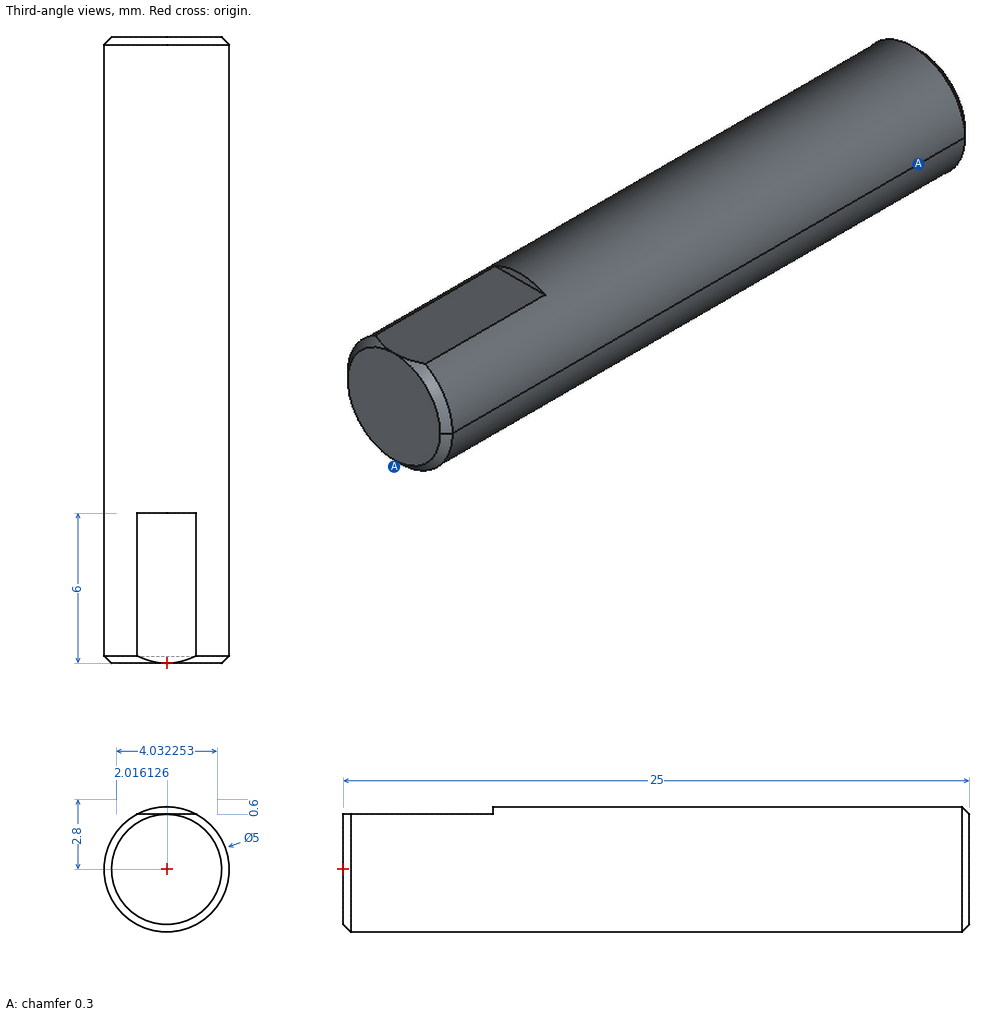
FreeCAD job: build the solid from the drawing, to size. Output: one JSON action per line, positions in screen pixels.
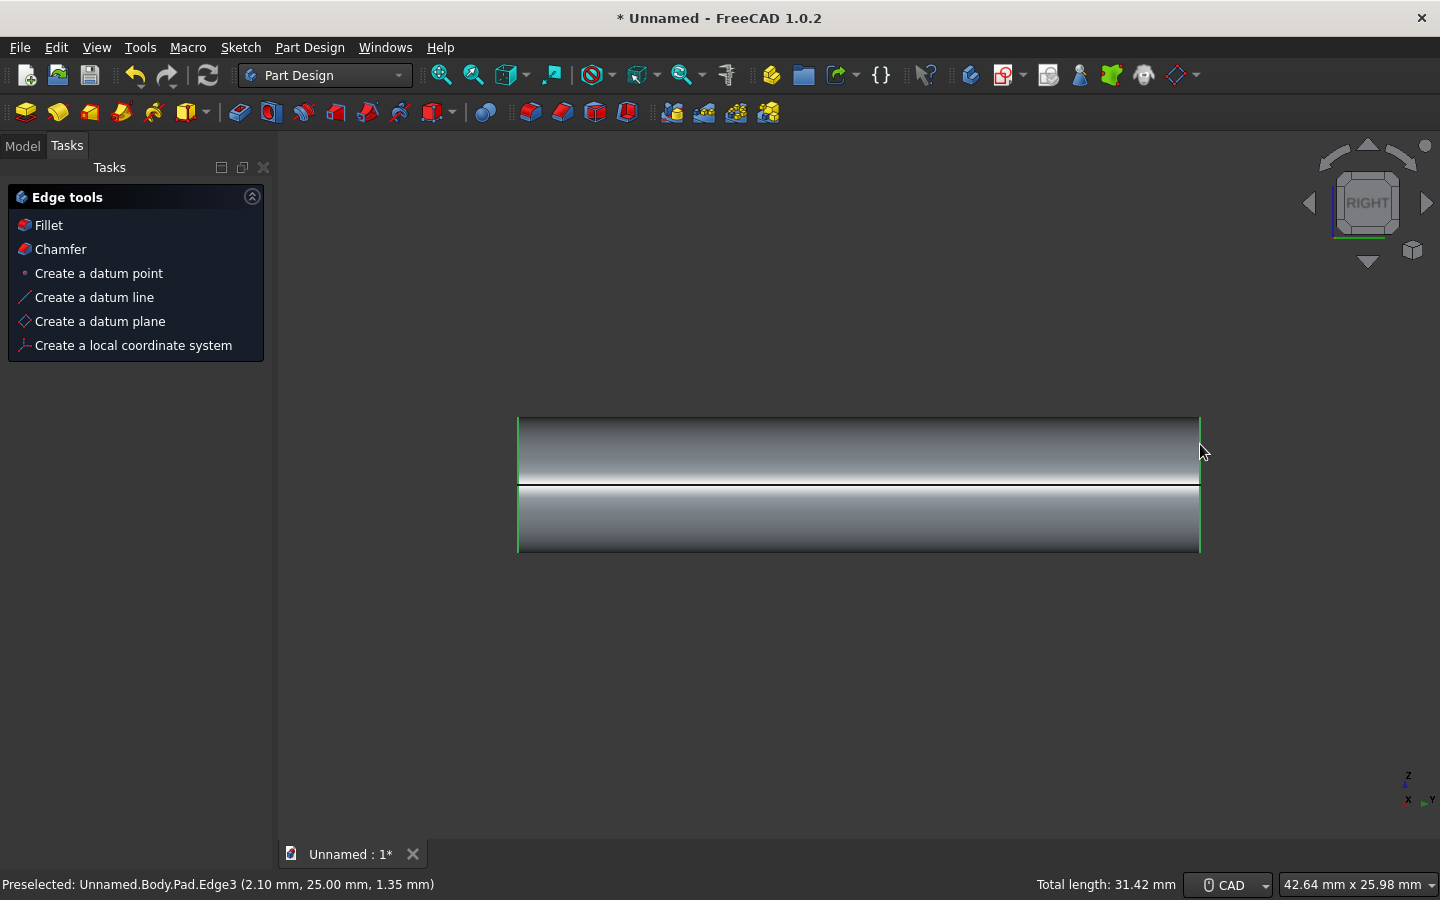
{"action": "left_click", "coordinate": [564, 112]}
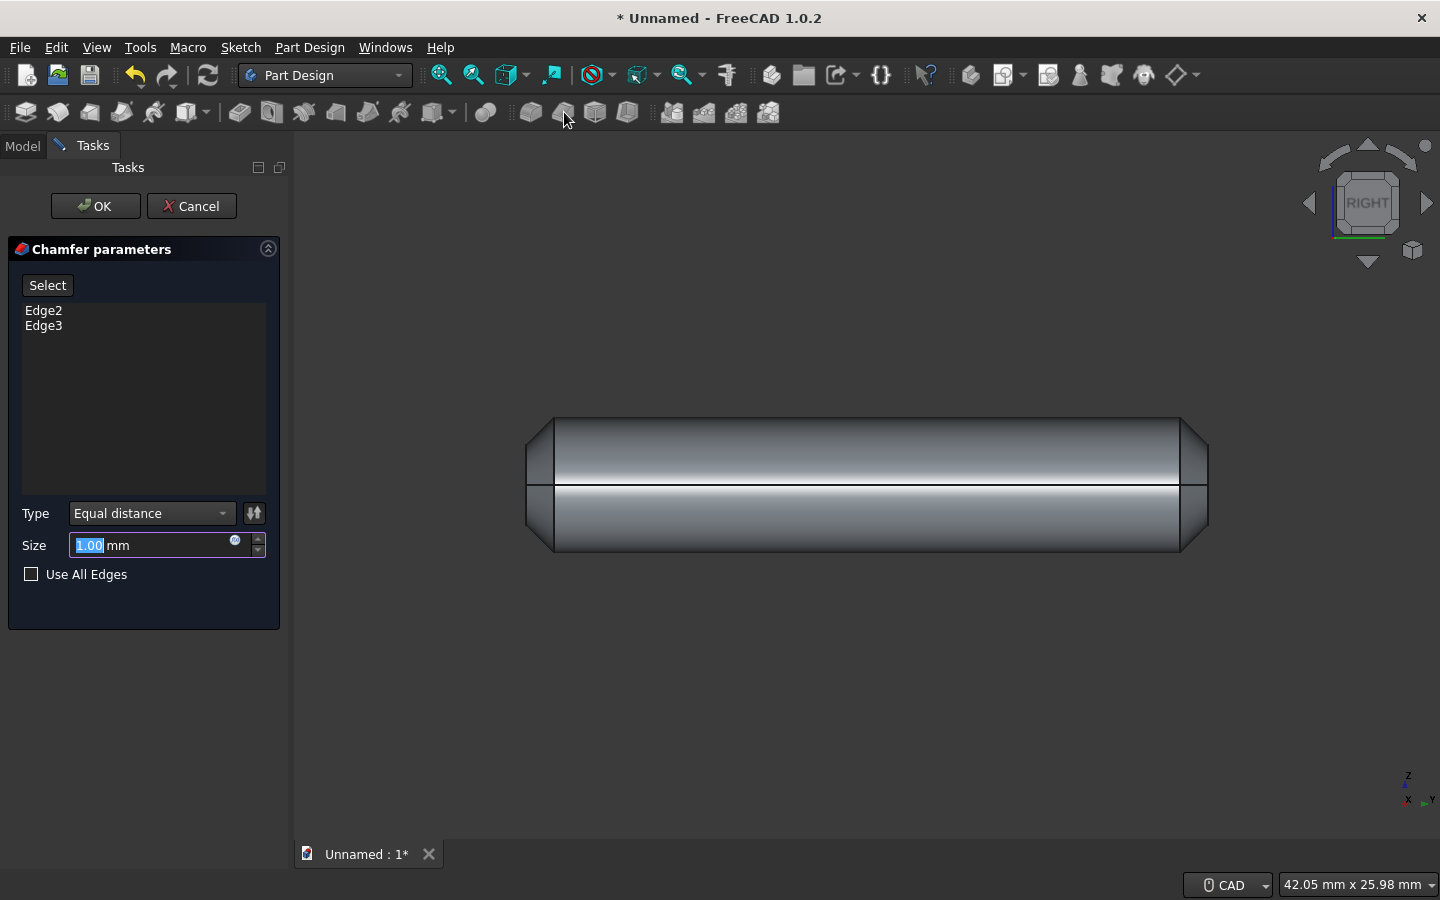
{"action": "type", "text": "0.3"}
{"action": "key", "text": "Tab"}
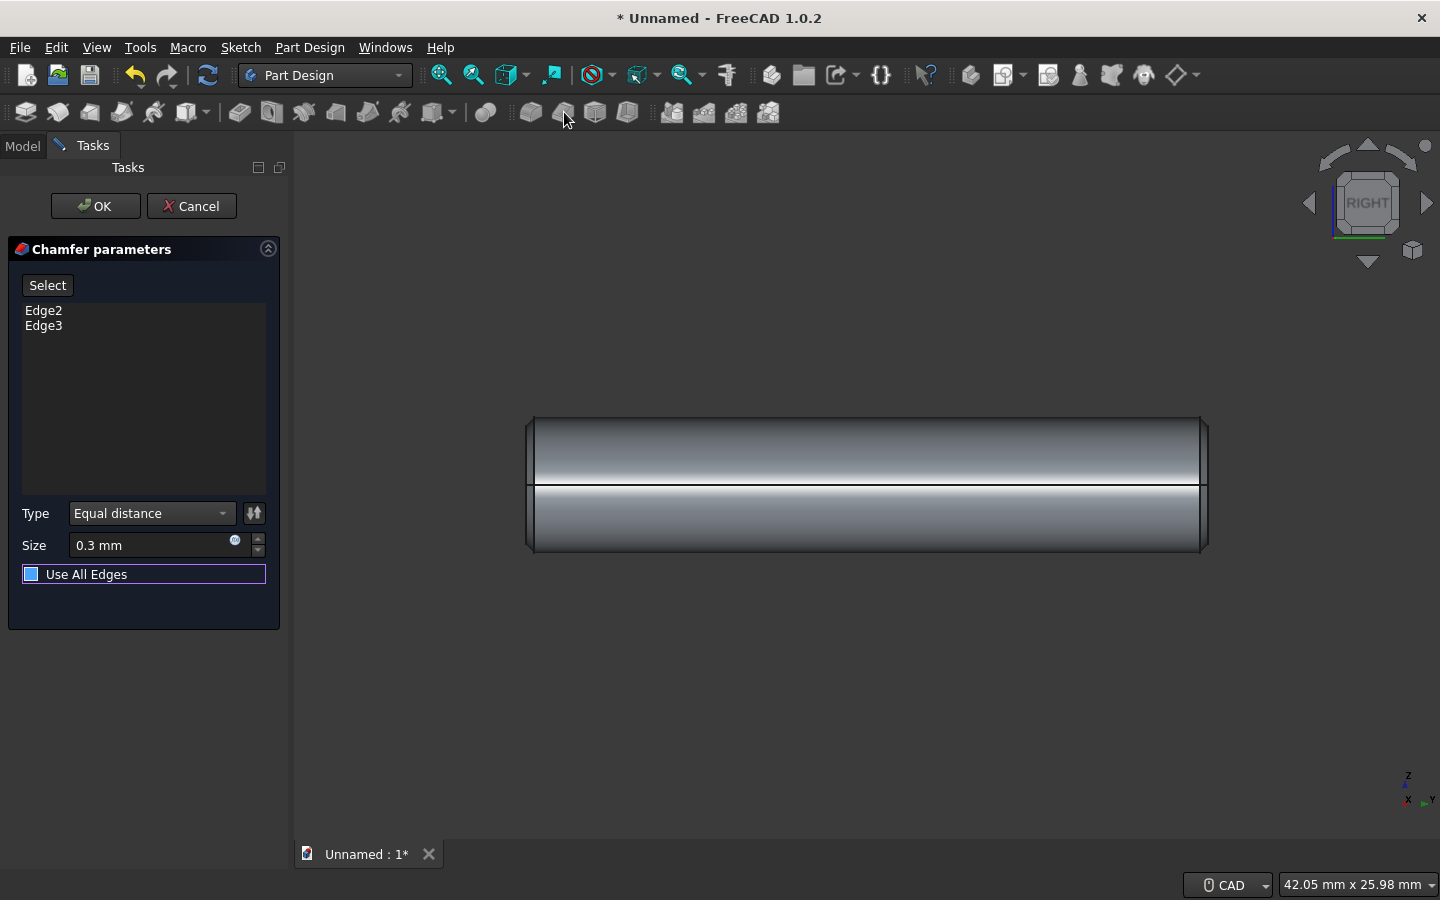
{"action": "left_click", "coordinate": [96, 206]}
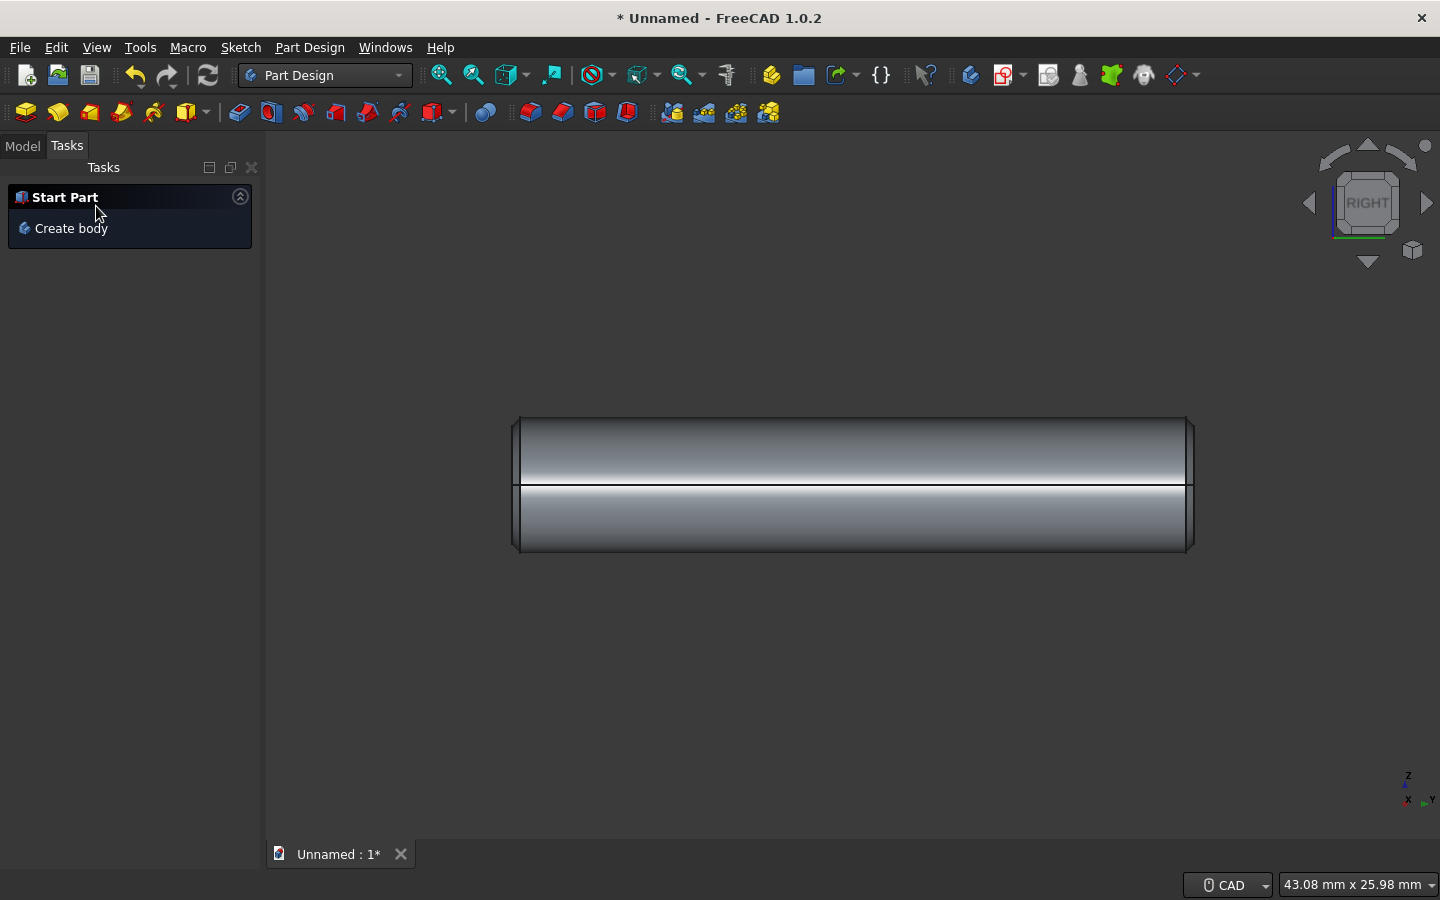
{"action": "left_click", "coordinate": [1004, 76]}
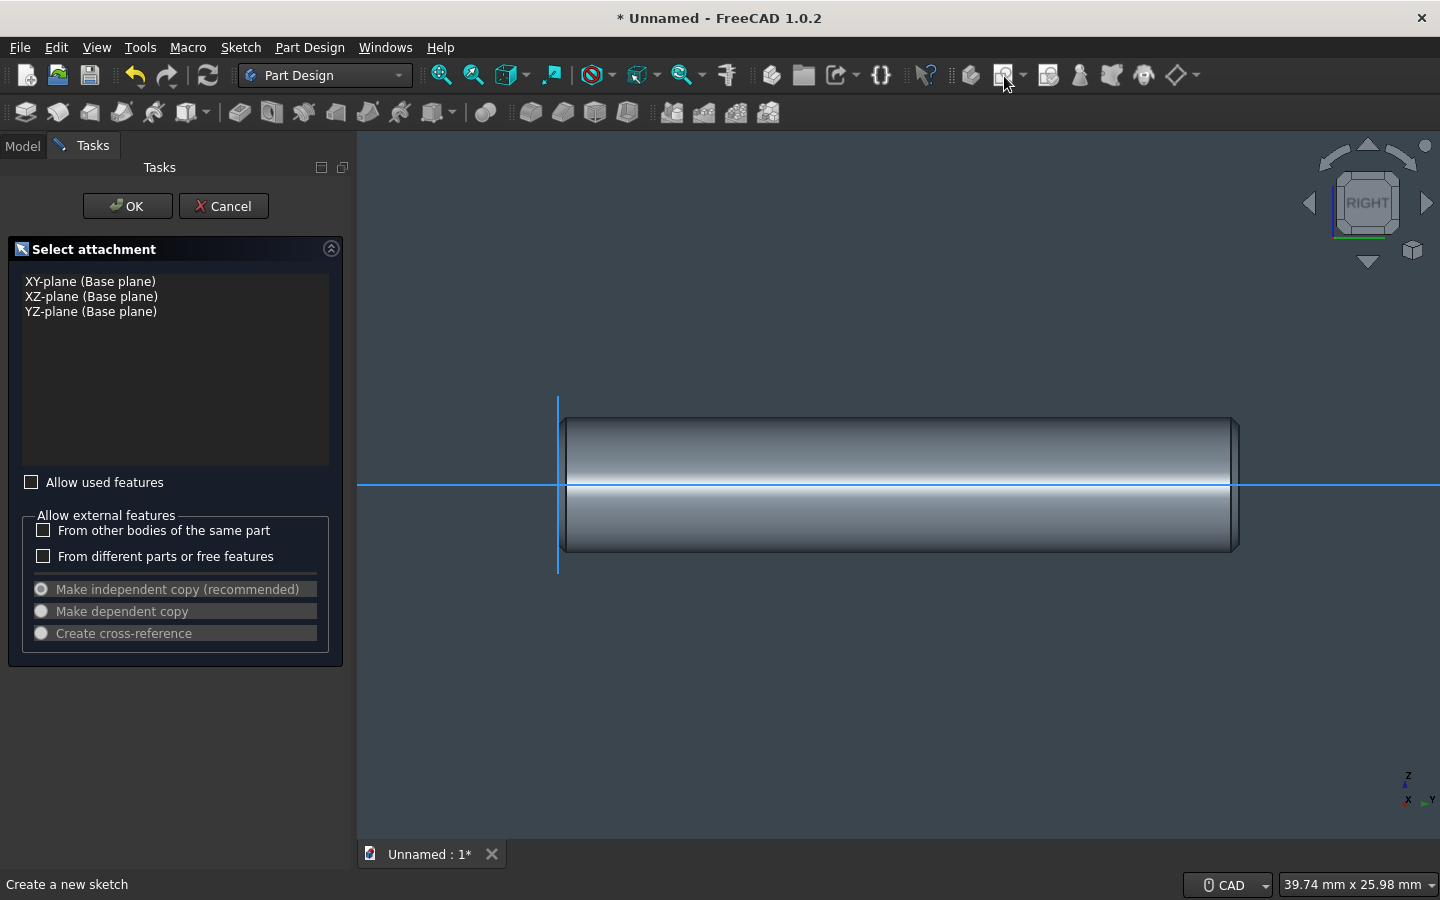
{"action": "left_click", "coordinate": [82, 296]}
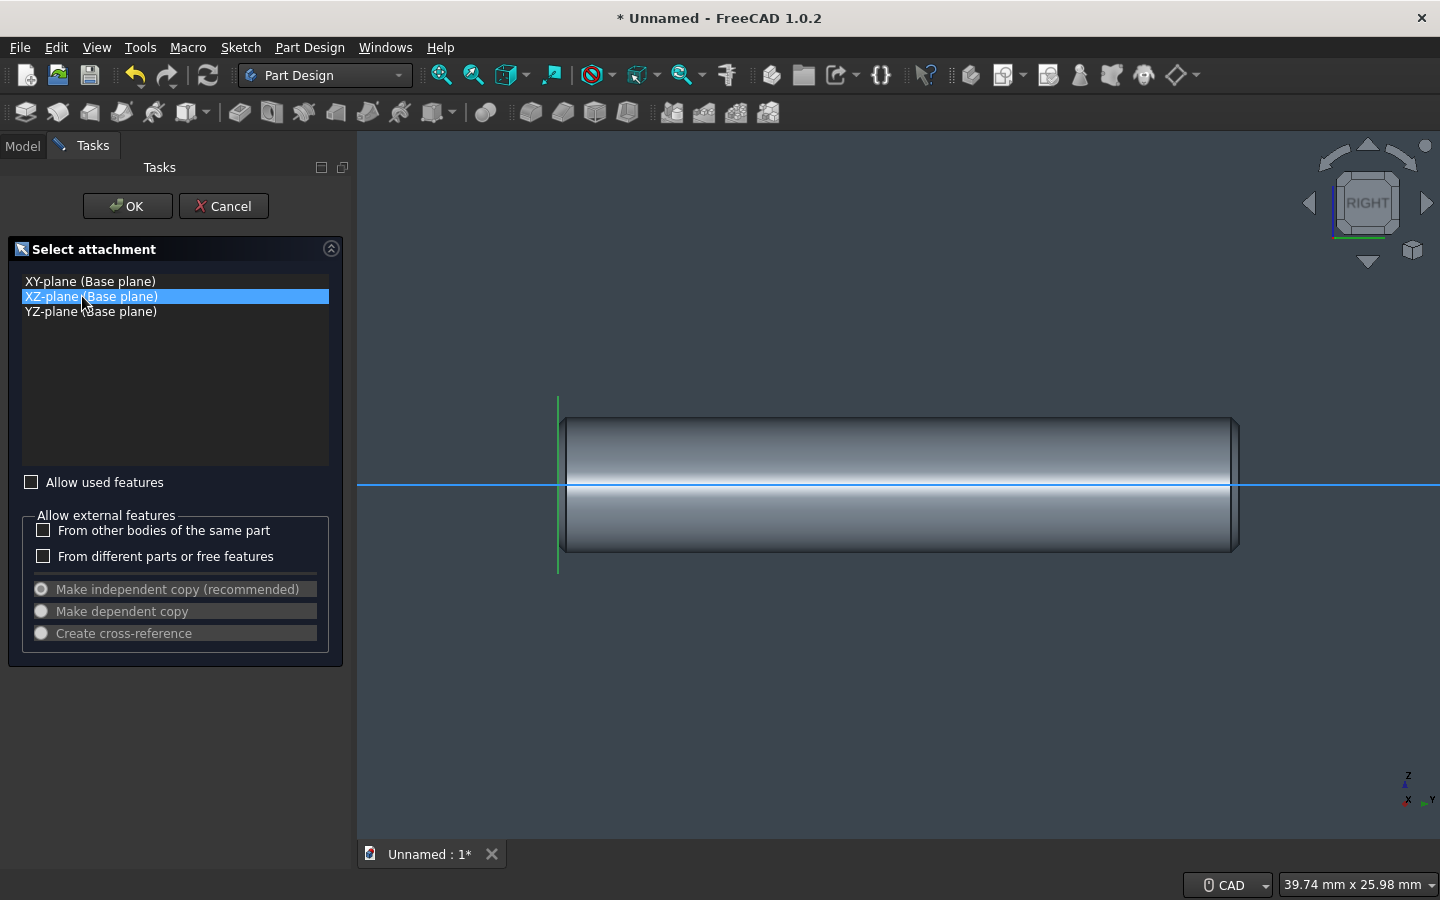
{"action": "left_click", "coordinate": [128, 206]}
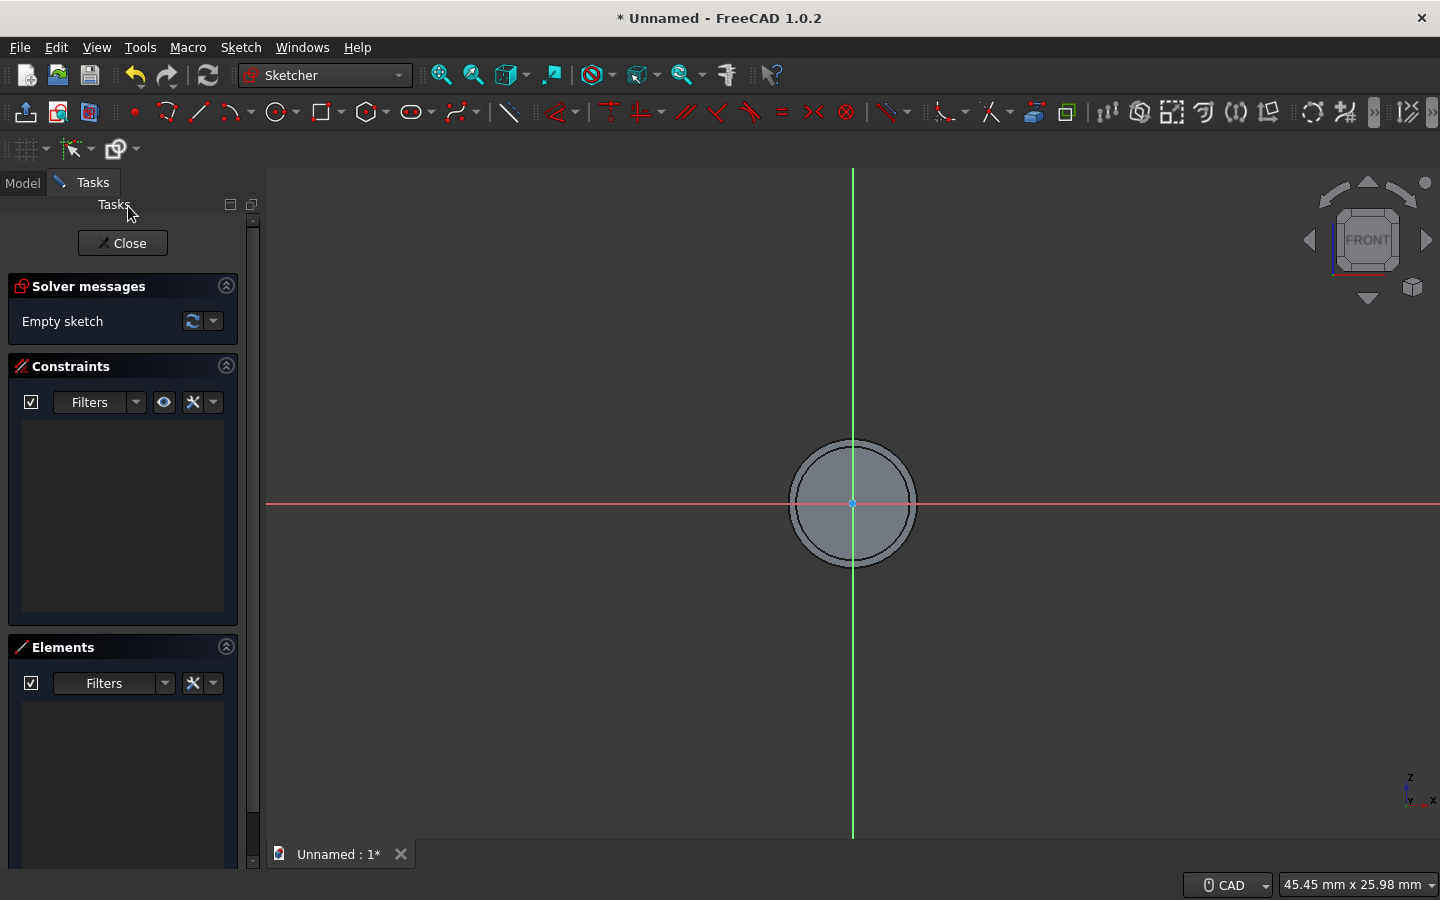
{"action": "scroll", "coordinate": [866, 460], "scroll_direction": "up", "scroll_amount": 9}